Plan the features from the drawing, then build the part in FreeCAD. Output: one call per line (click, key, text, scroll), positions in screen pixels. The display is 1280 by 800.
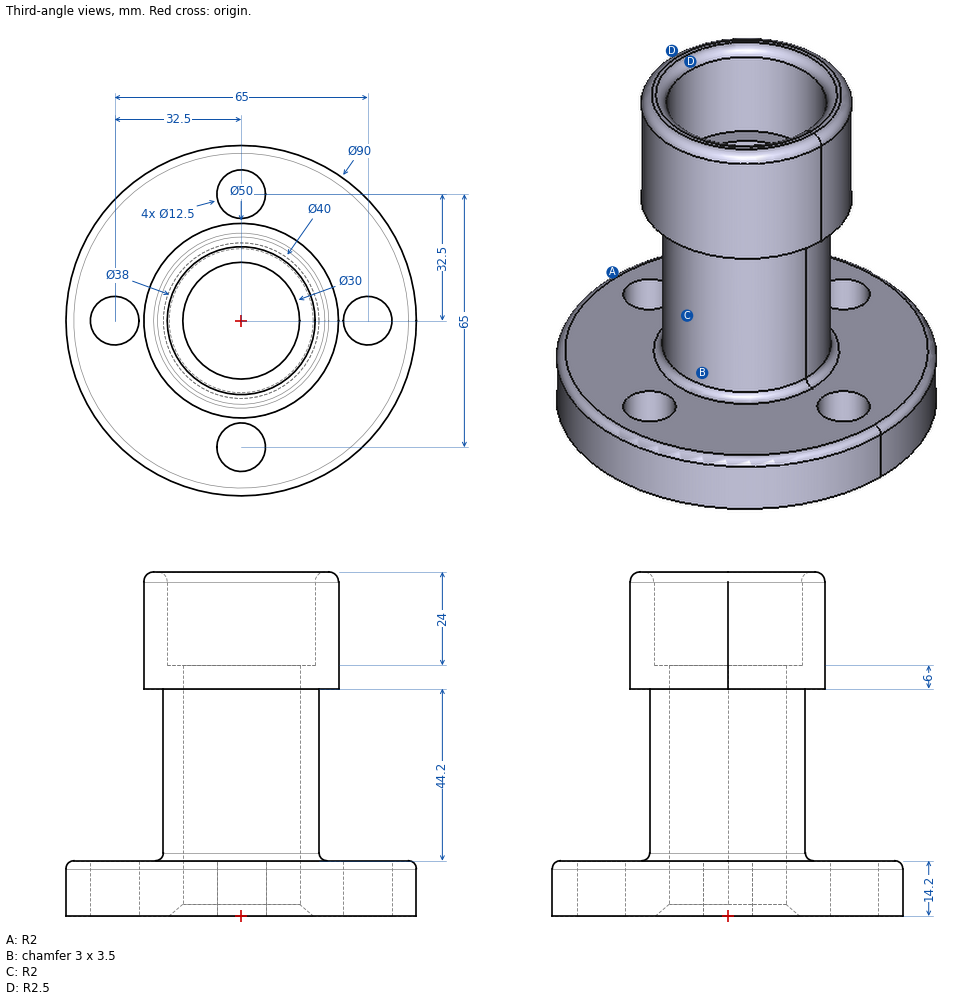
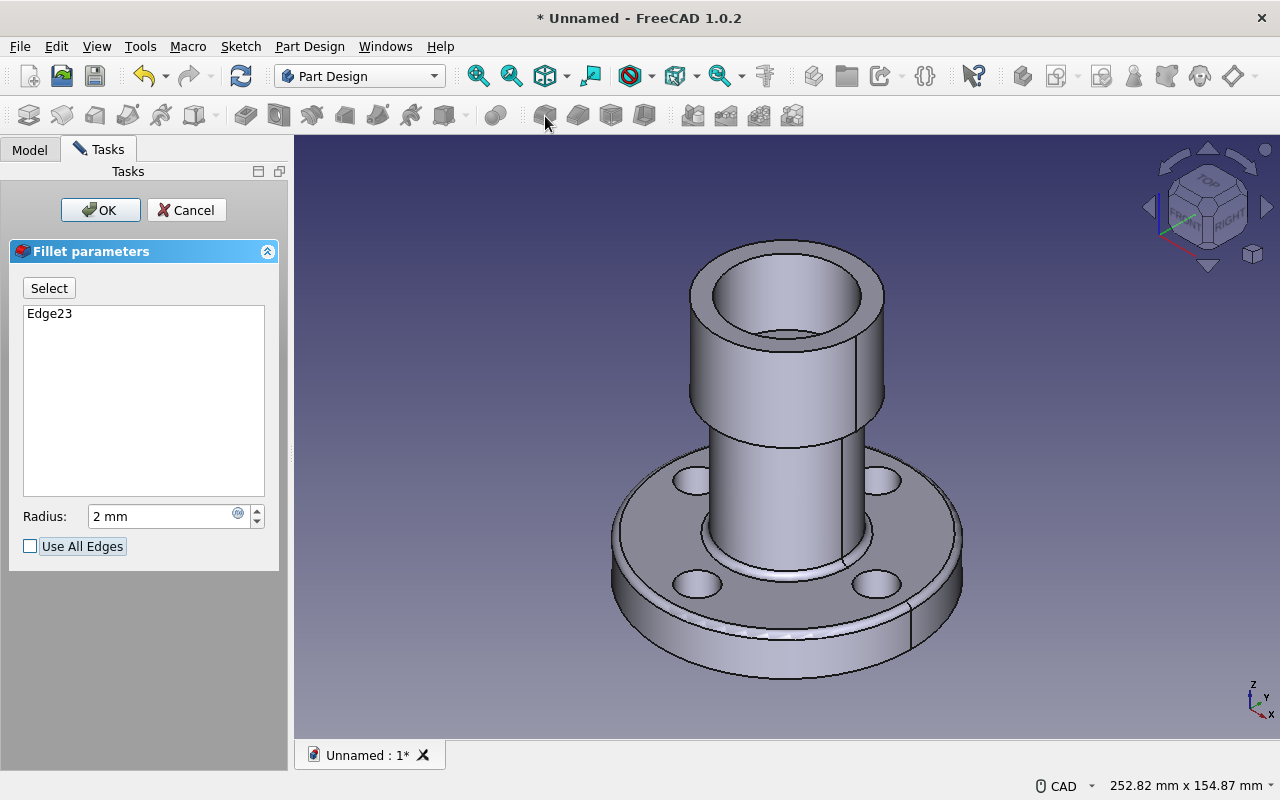
click(101, 210)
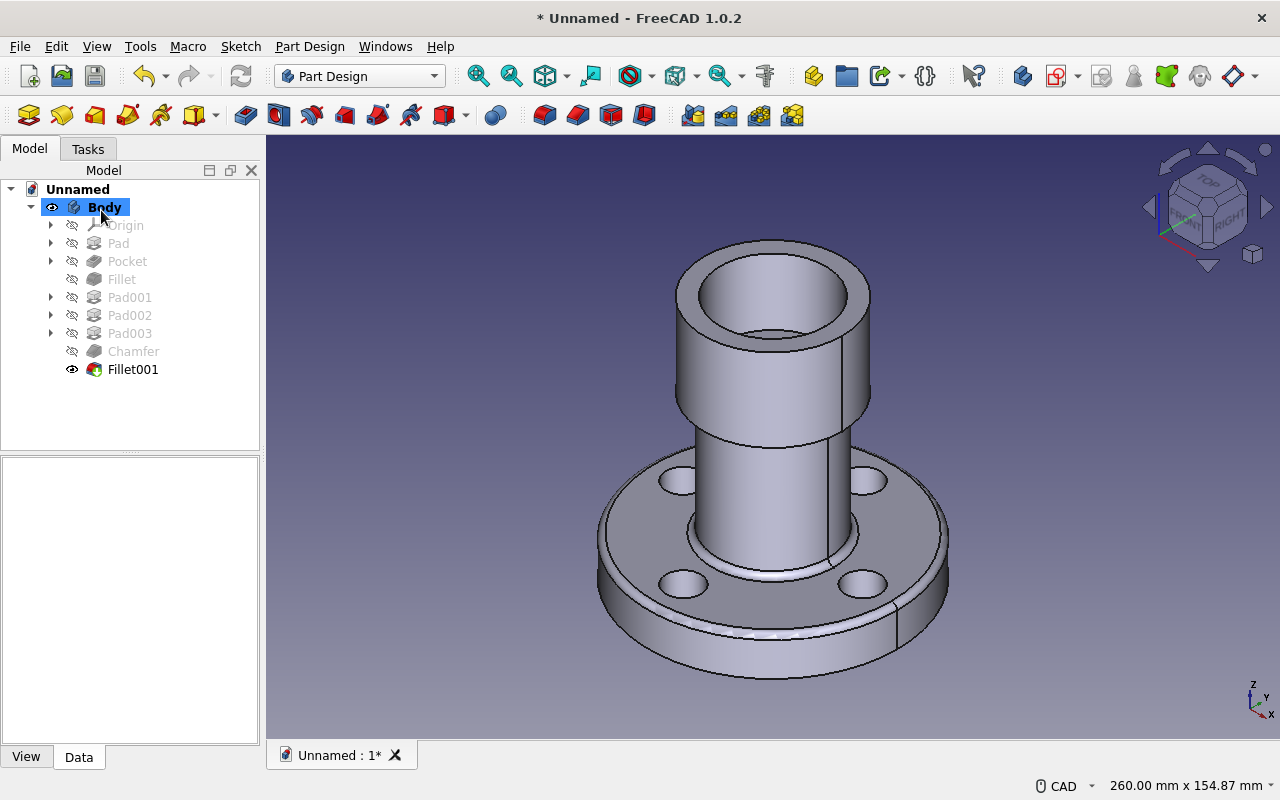
click(686, 321)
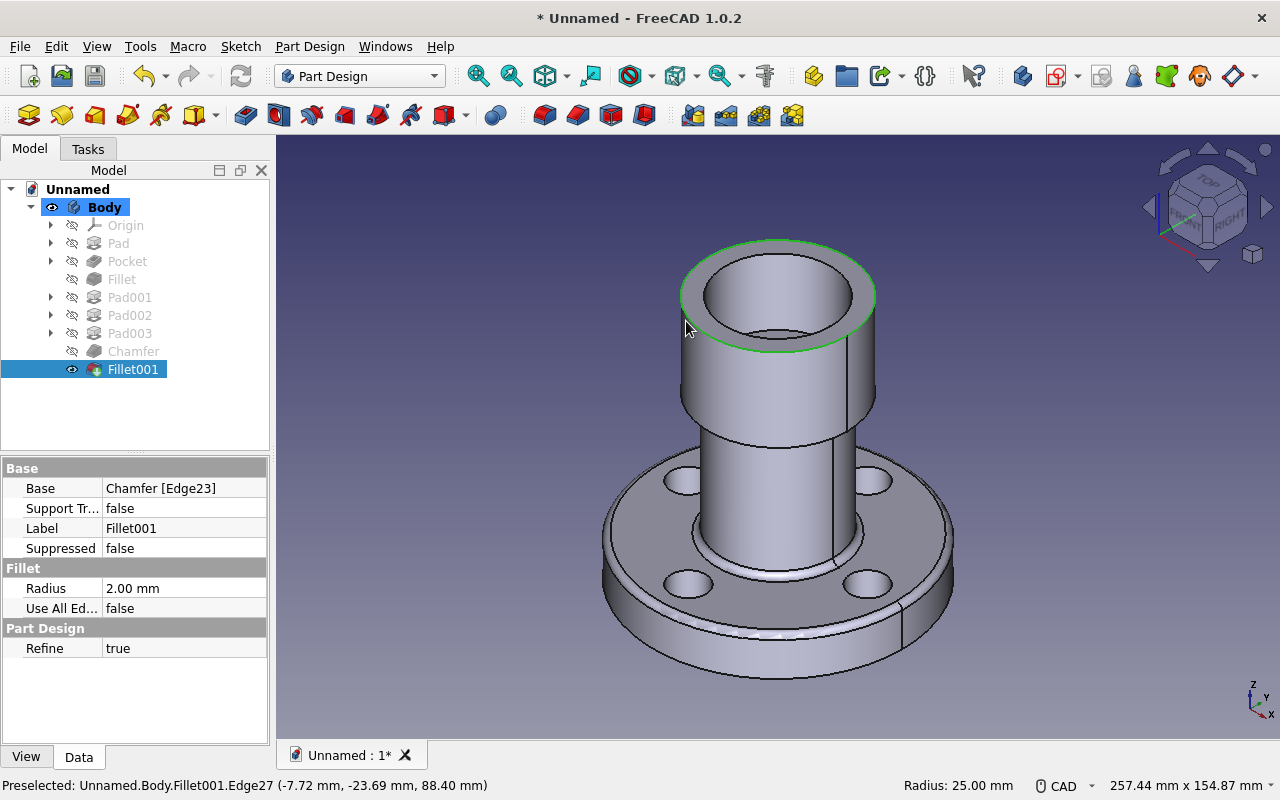
click(726, 265, ctrl)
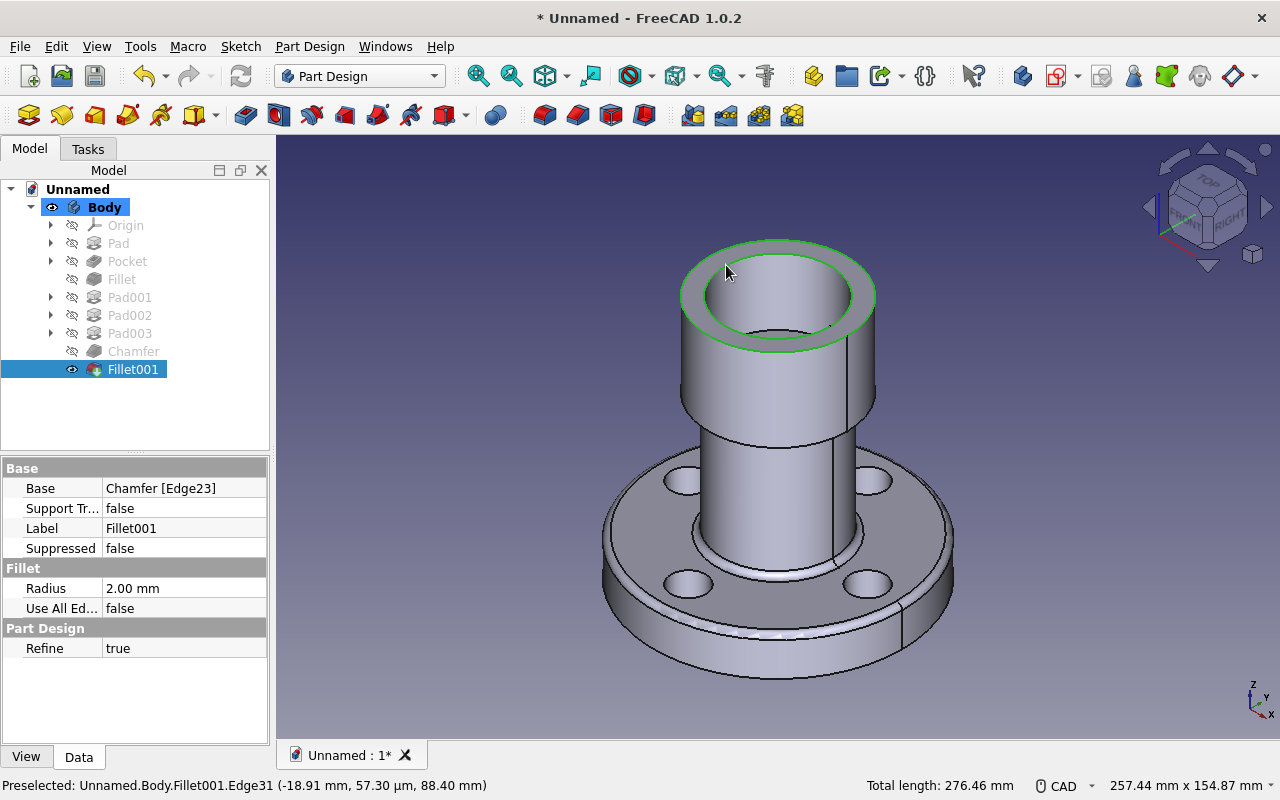
click(545, 116)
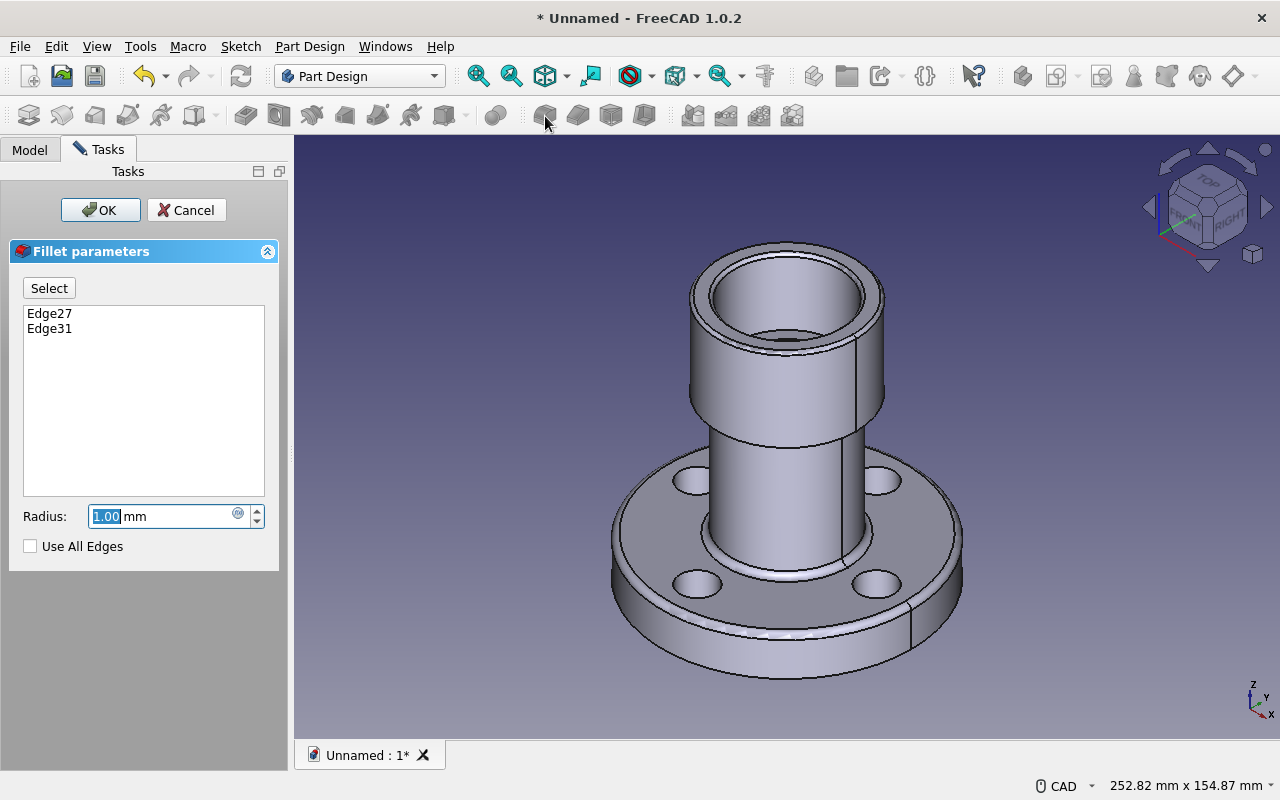
text(2.5)
key(Tab)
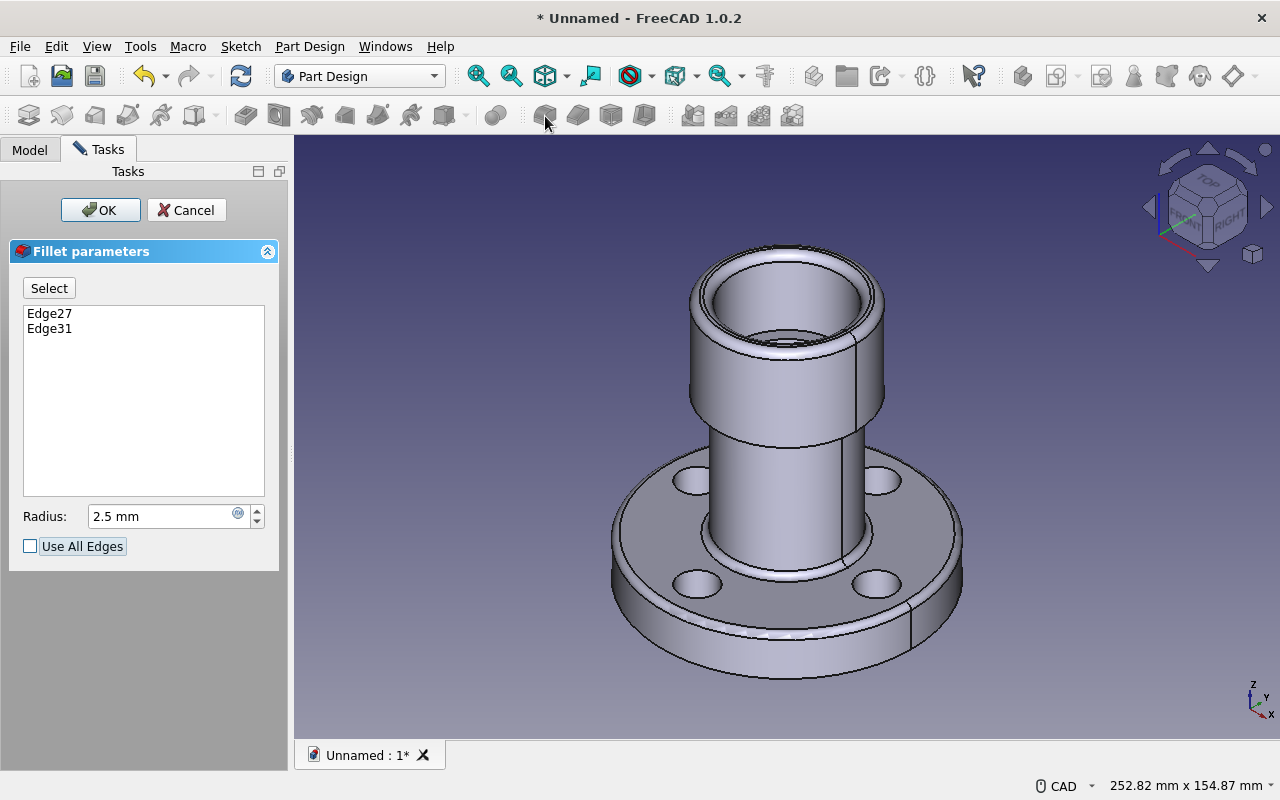
click(101, 210)